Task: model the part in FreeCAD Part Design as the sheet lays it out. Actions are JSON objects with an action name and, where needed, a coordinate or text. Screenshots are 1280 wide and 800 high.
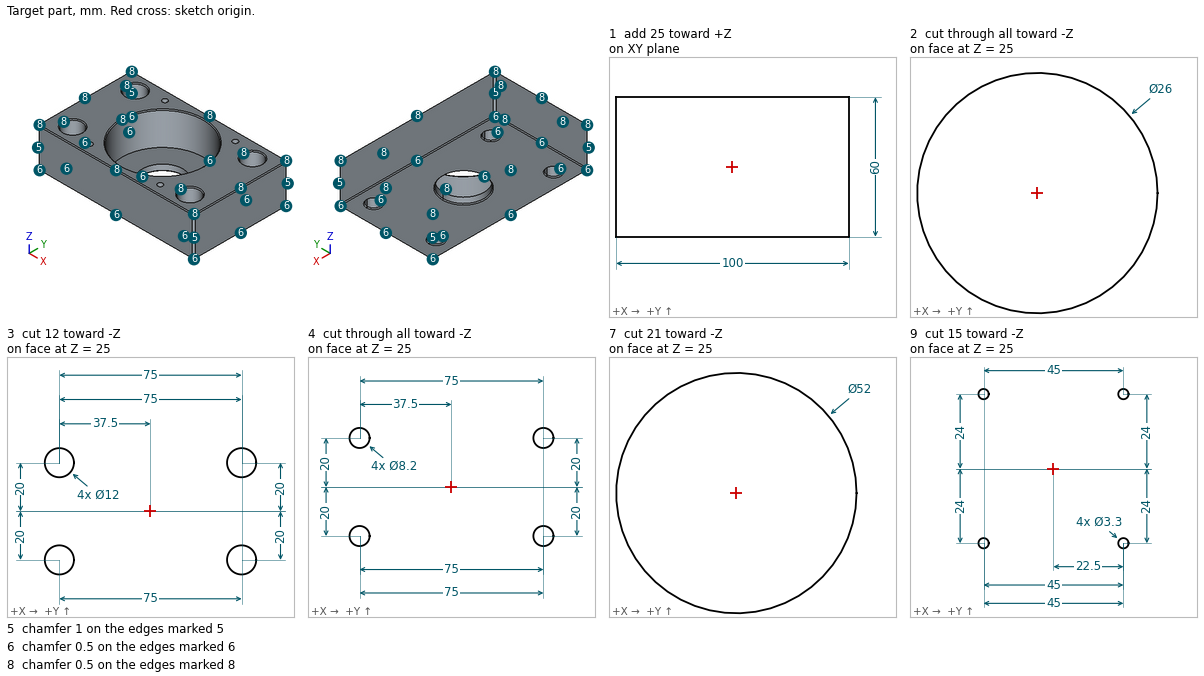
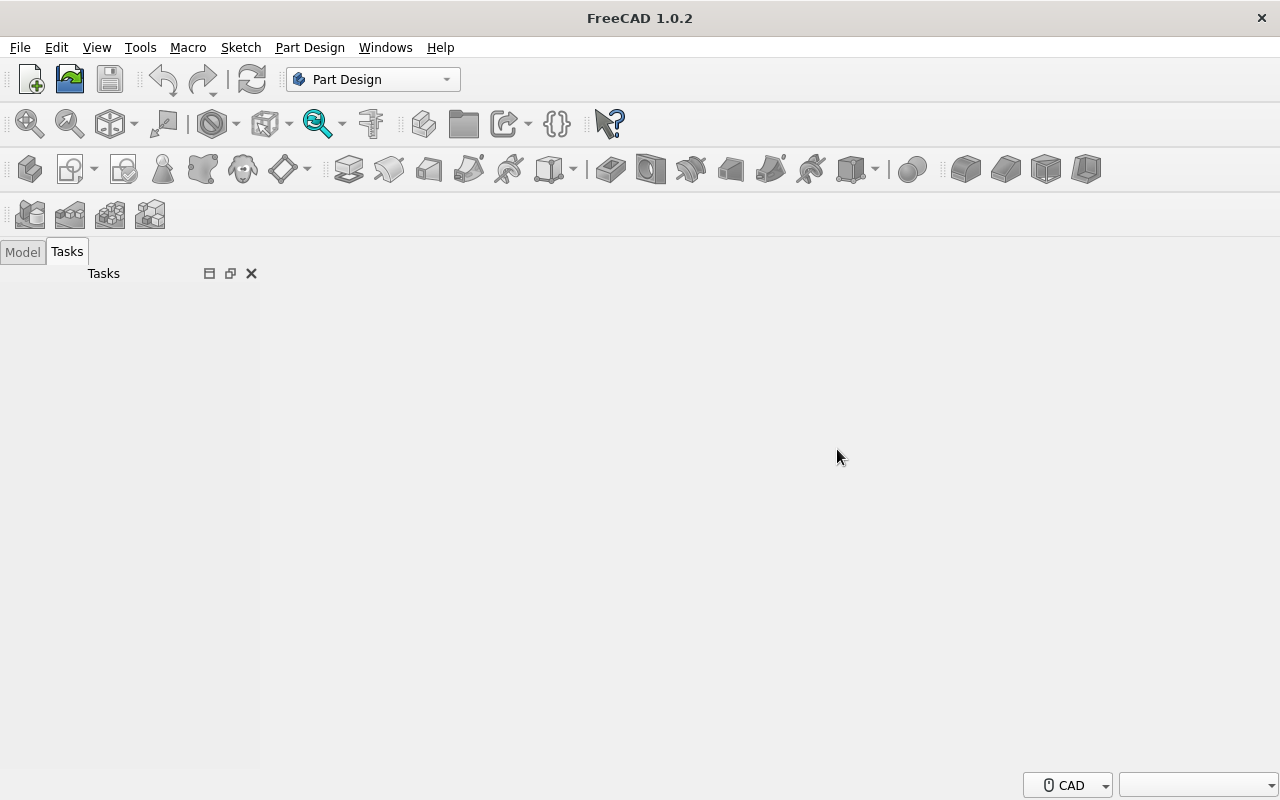
{"action": "left_click", "coordinate": [30, 80]}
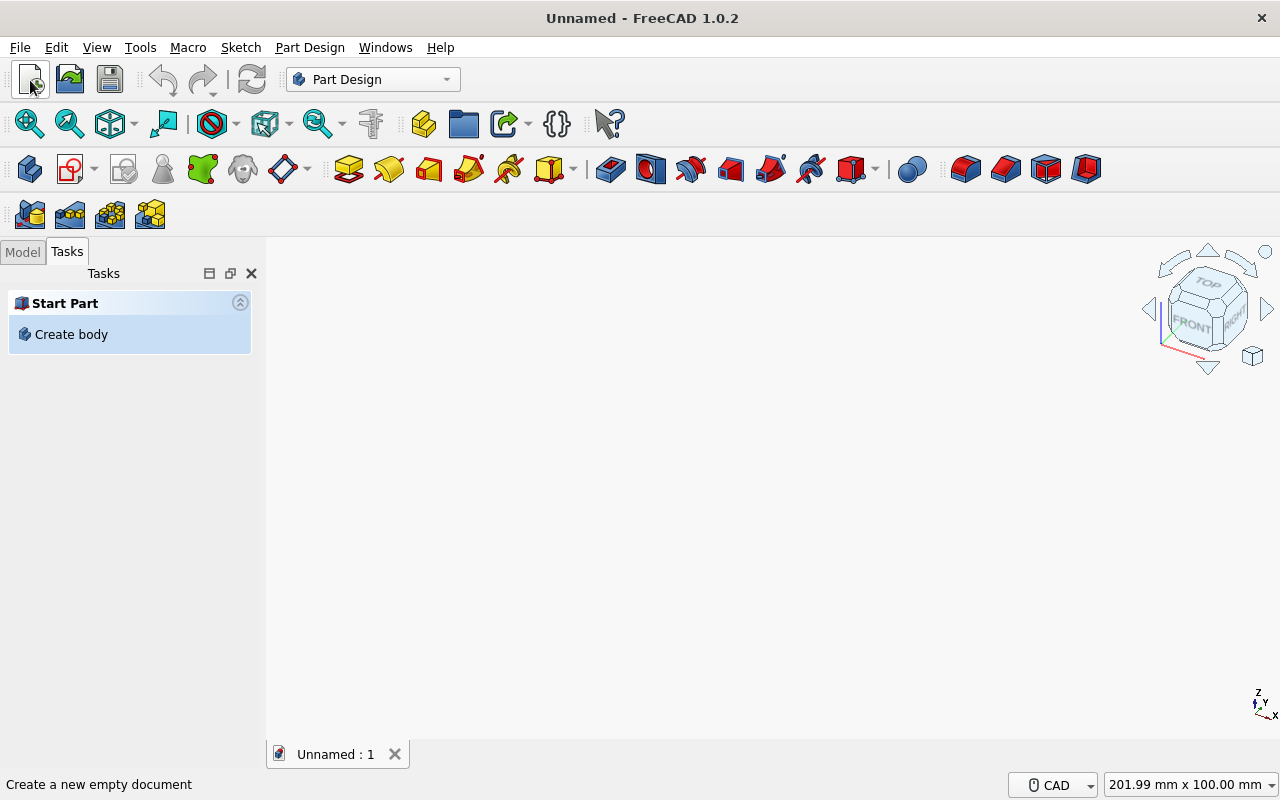
{"action": "left_click", "coordinate": [70, 170]}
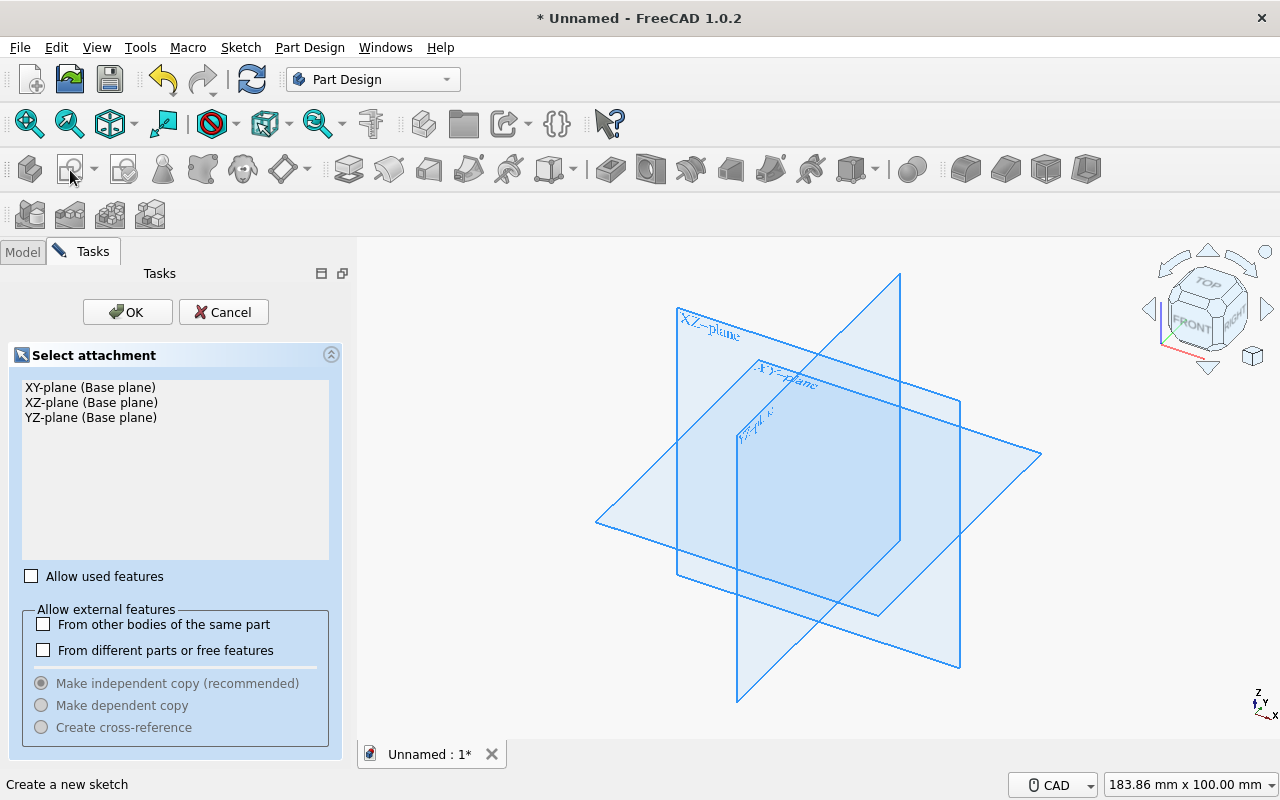
{"action": "left_click", "coordinate": [82, 388]}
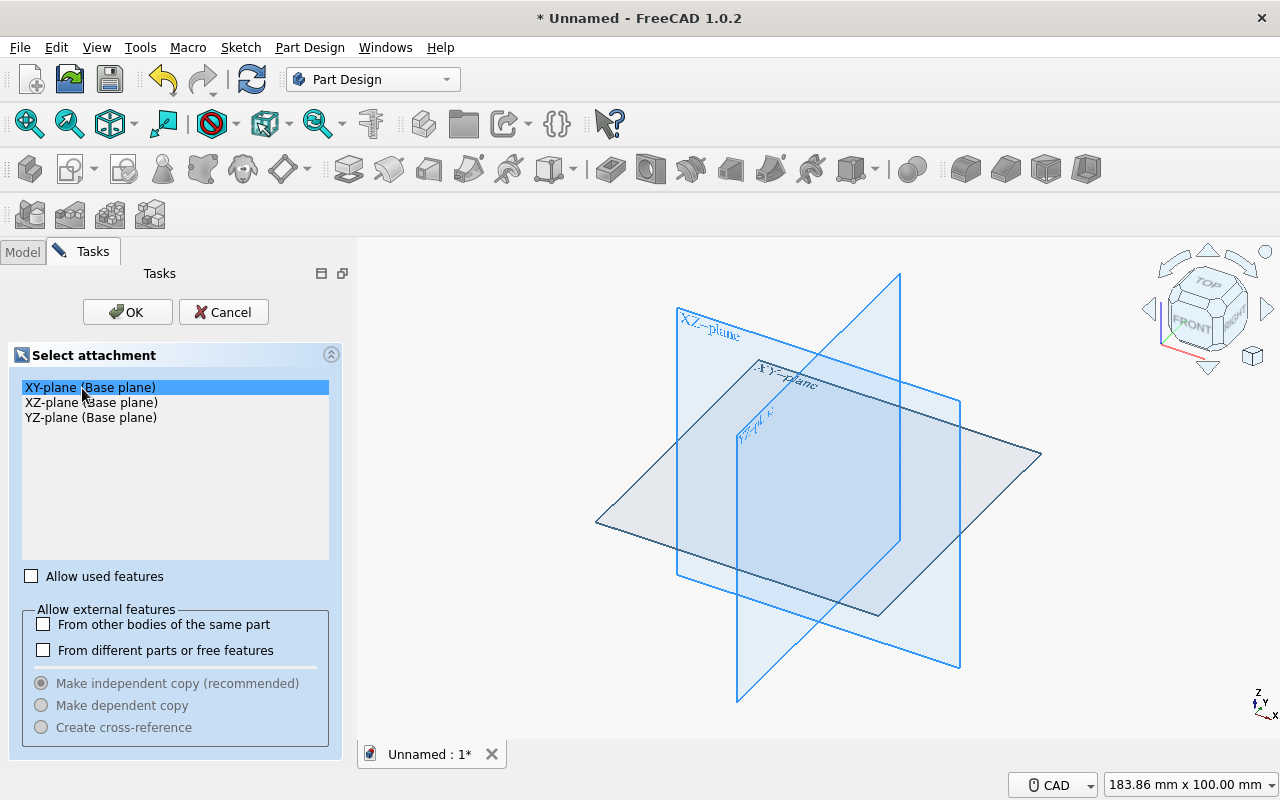
{"action": "left_click", "coordinate": [128, 312]}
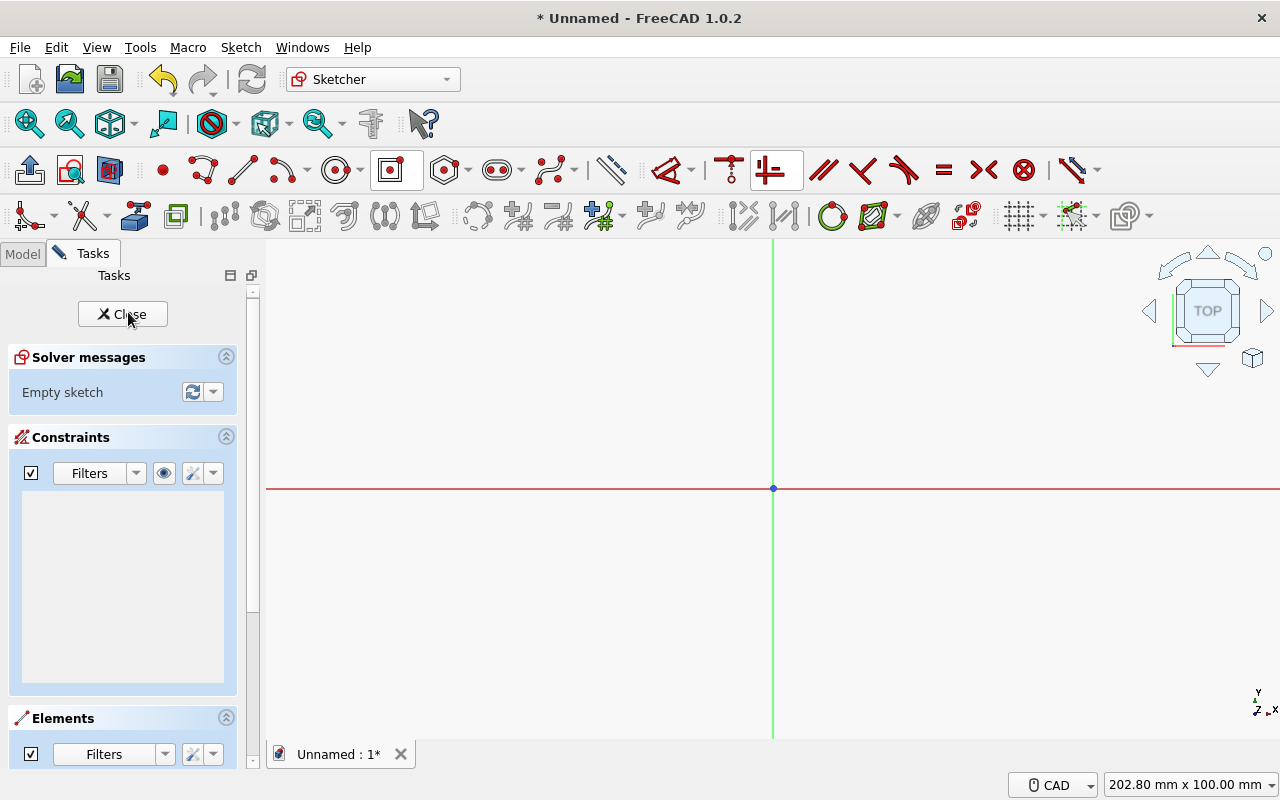
{"action": "left_click", "coordinate": [390, 170]}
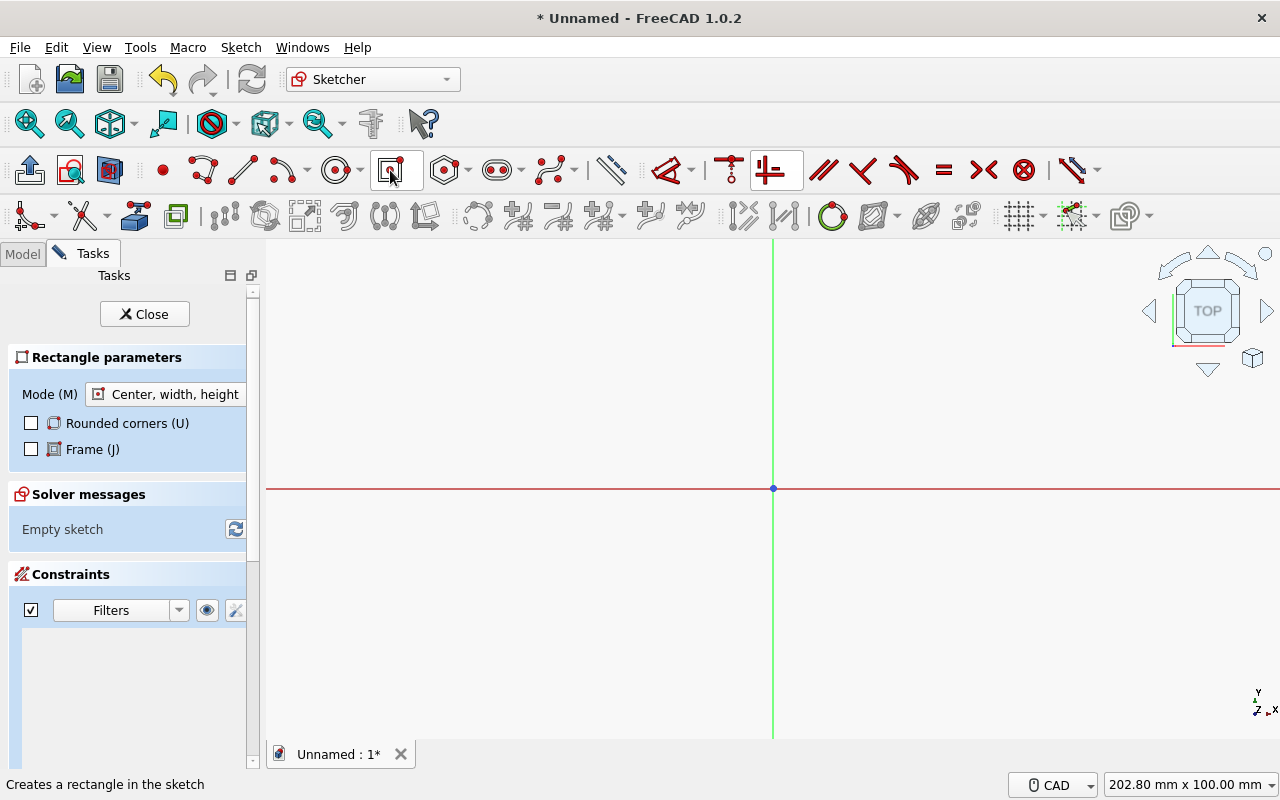
{"action": "left_click", "coordinate": [773, 489]}
{"action": "mouse_move", "coordinate": [1023, 339]}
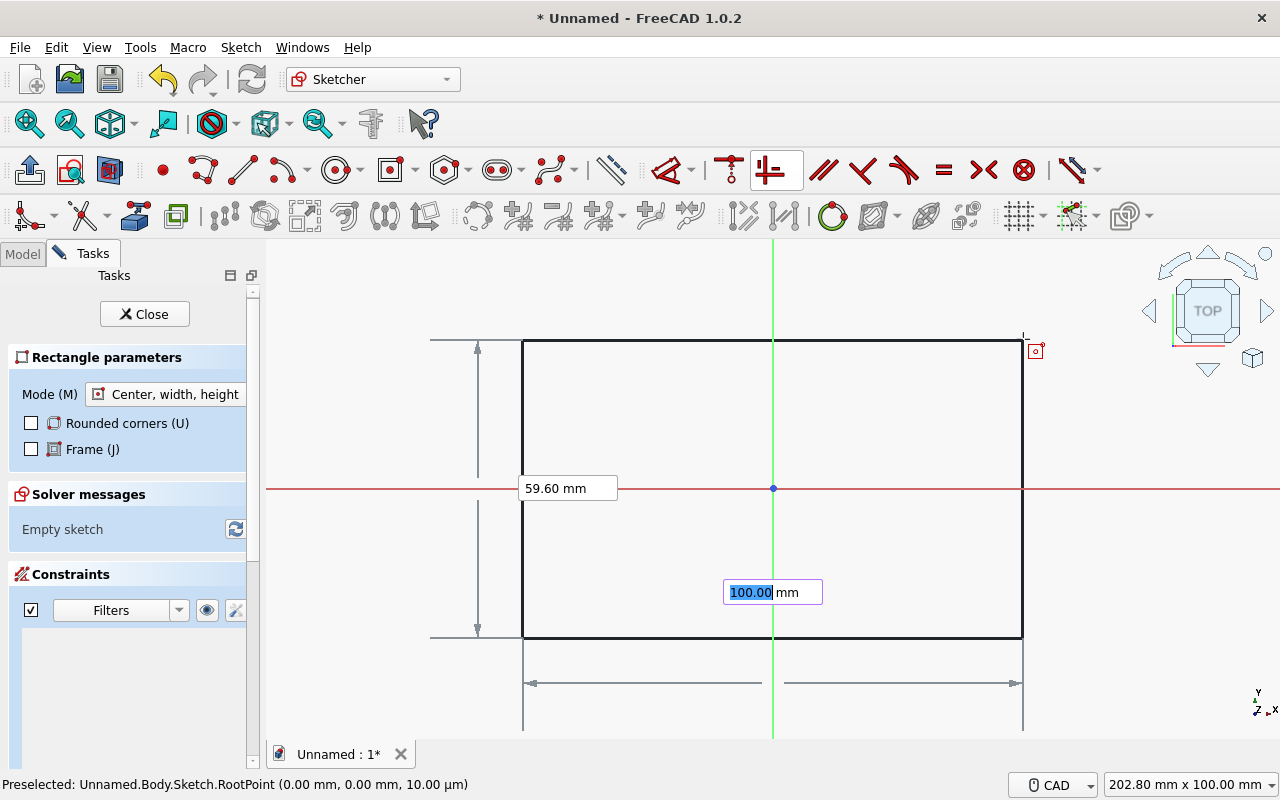
{"action": "type", "text": "100"}
{"action": "key", "text": "Tab"}
{"action": "type", "text": "60"}
{"action": "key", "text": "Return"}
{"action": "key", "text": "Escape"}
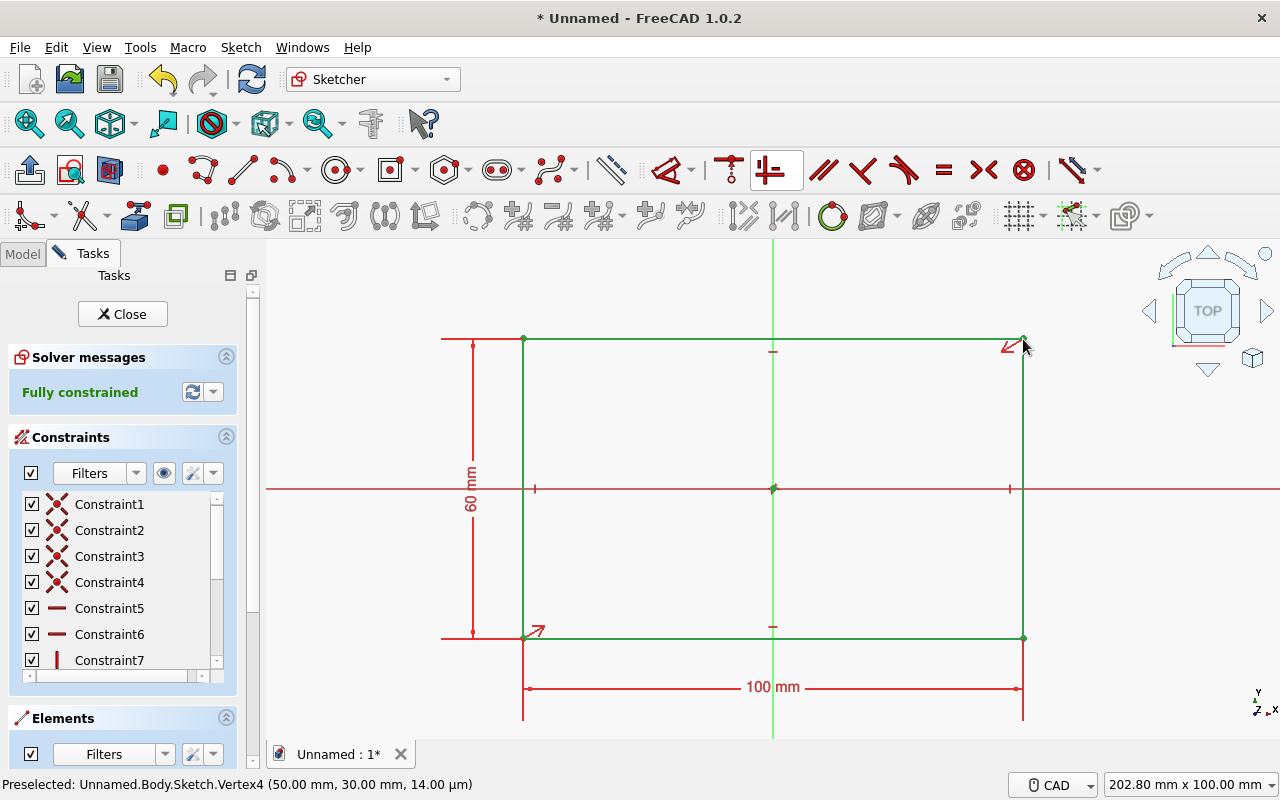
{"action": "left_click", "coordinate": [123, 314]}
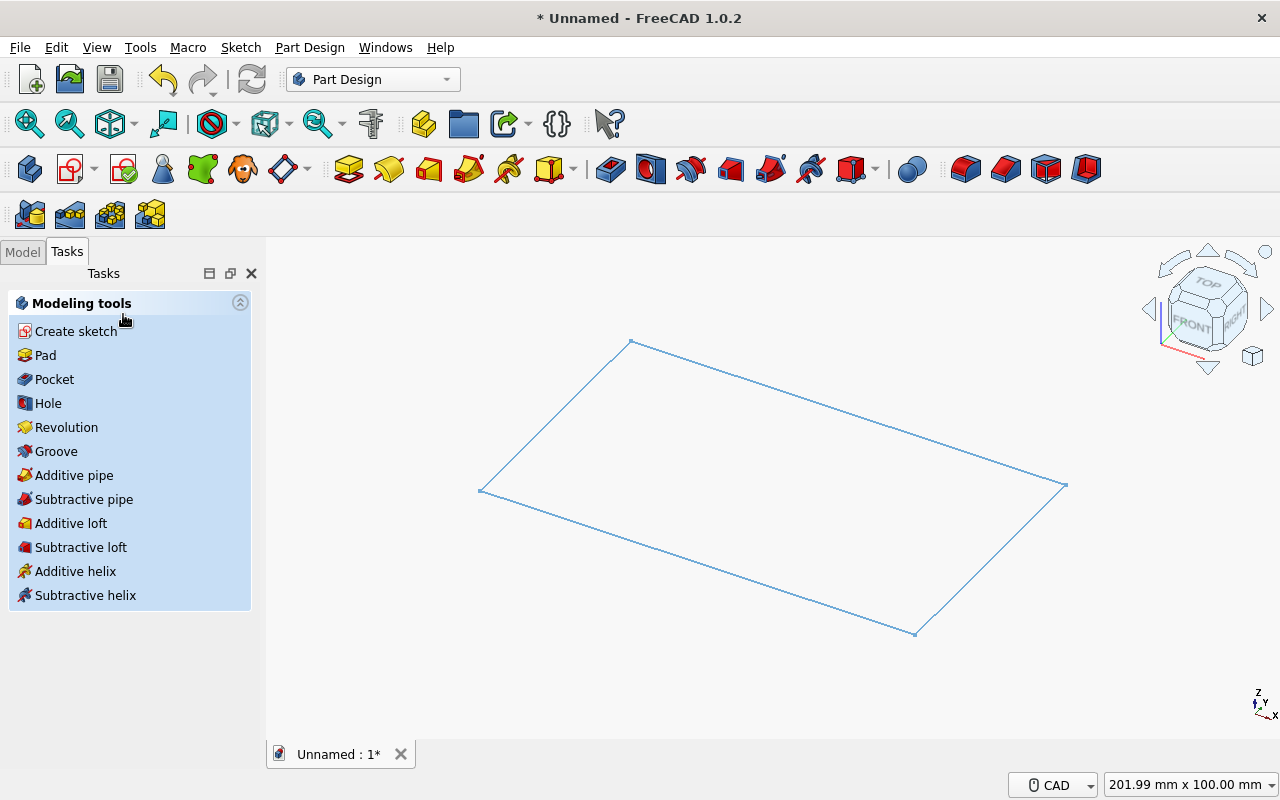
{"action": "left_click", "coordinate": [350, 170]}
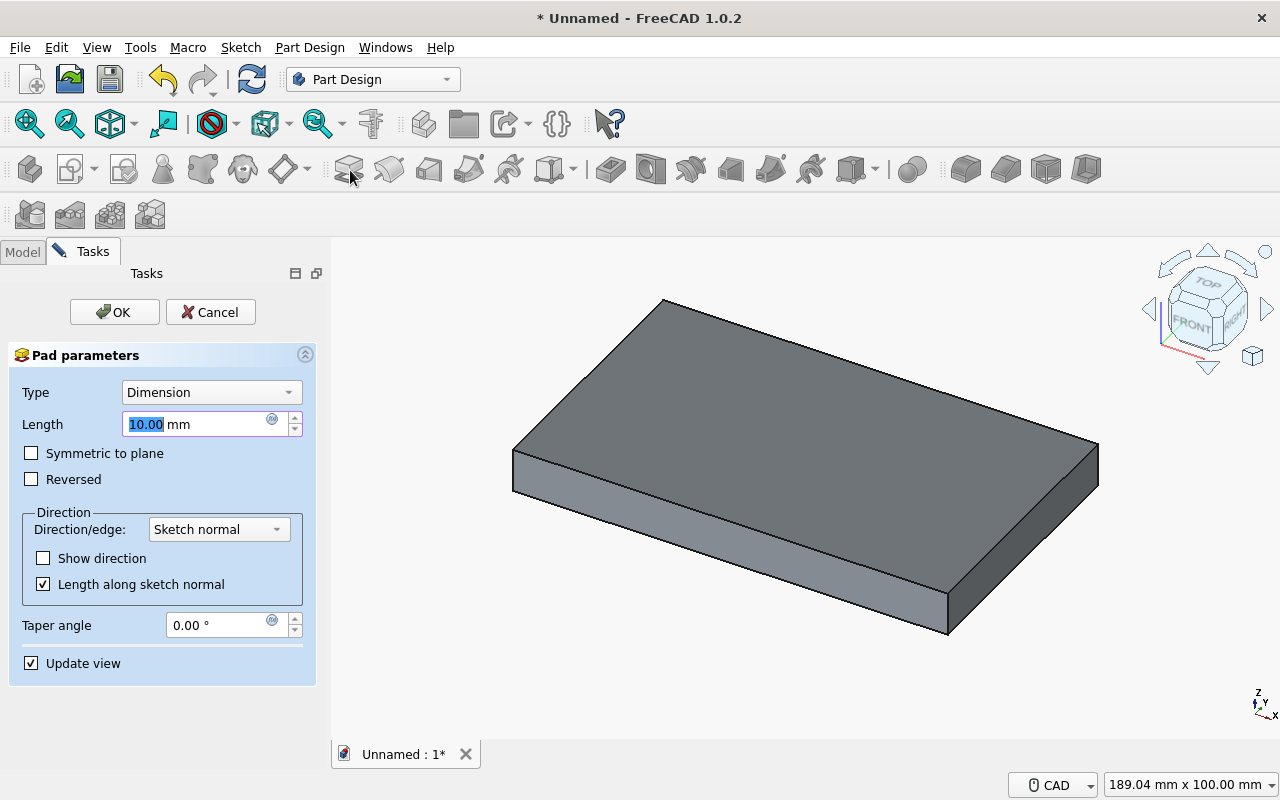
{"action": "type", "text": "25"}
{"action": "key", "text": "Tab"}